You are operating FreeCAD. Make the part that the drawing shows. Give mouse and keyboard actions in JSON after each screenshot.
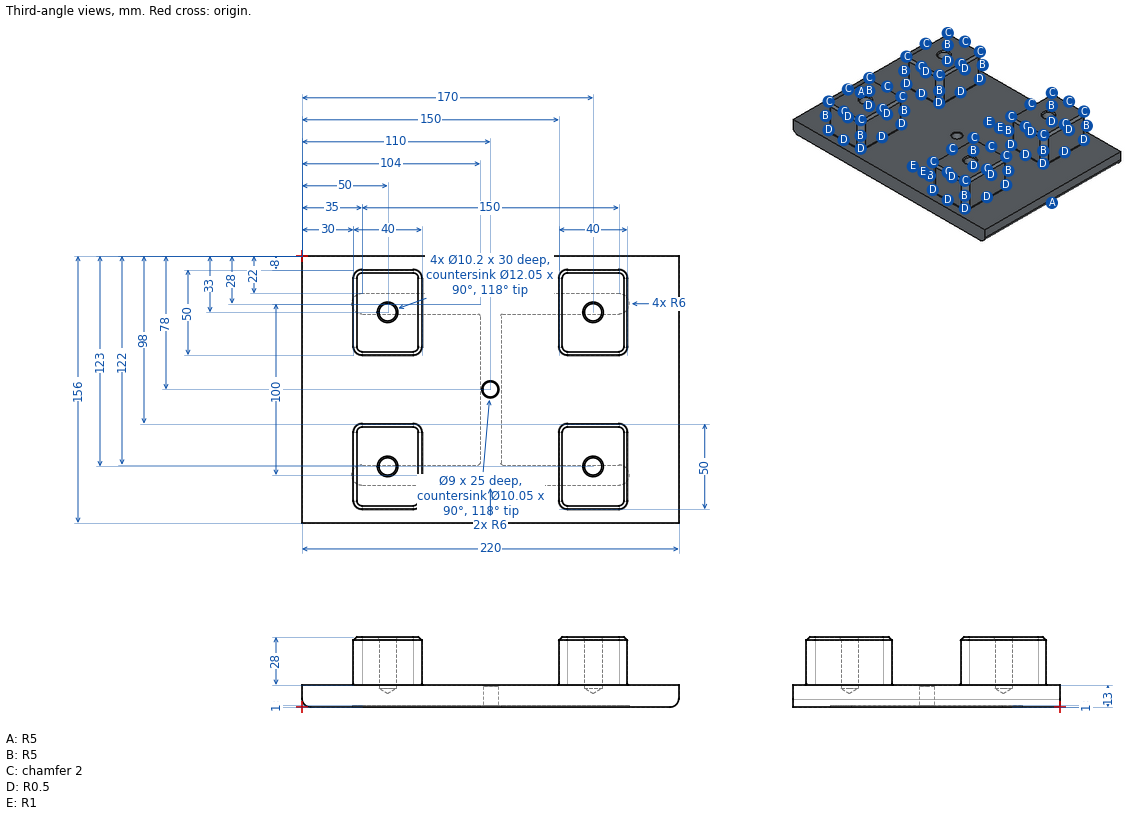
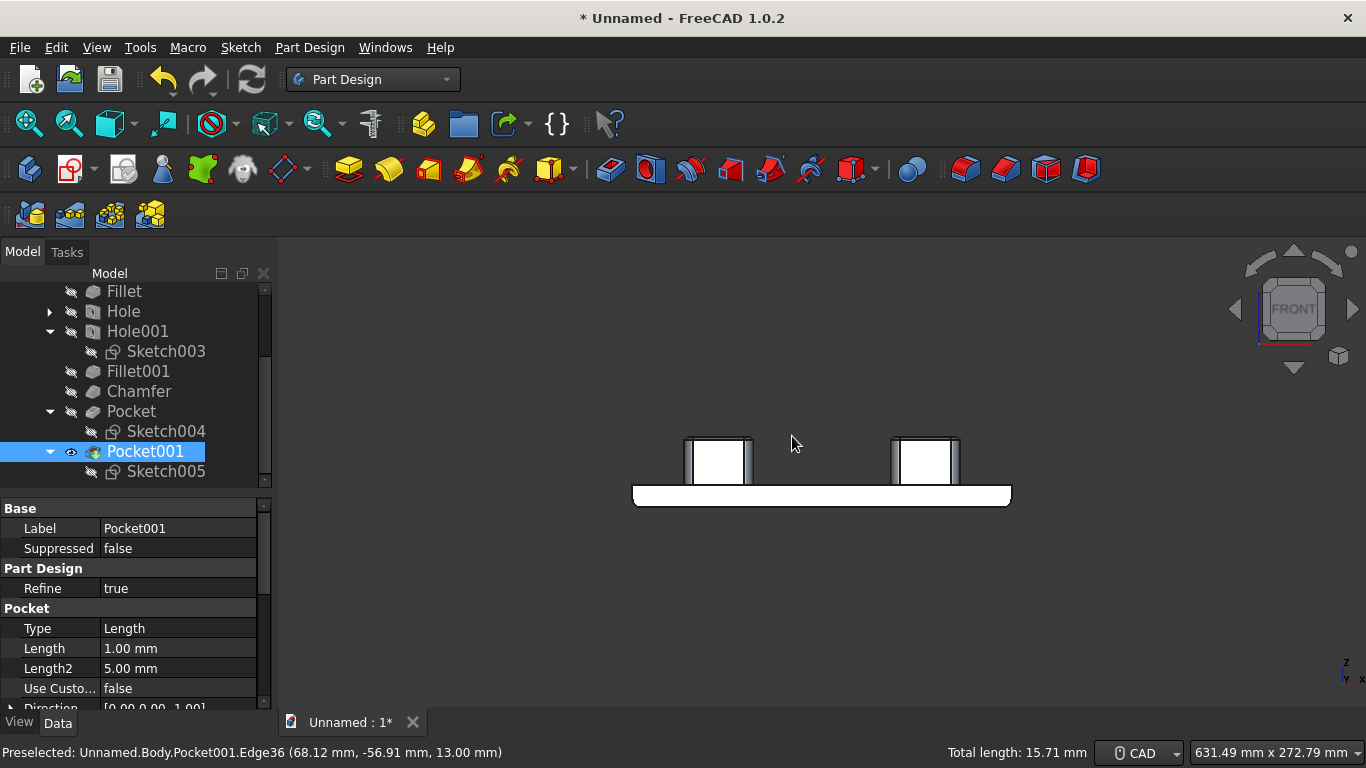
{"action": "key", "text": "v f"}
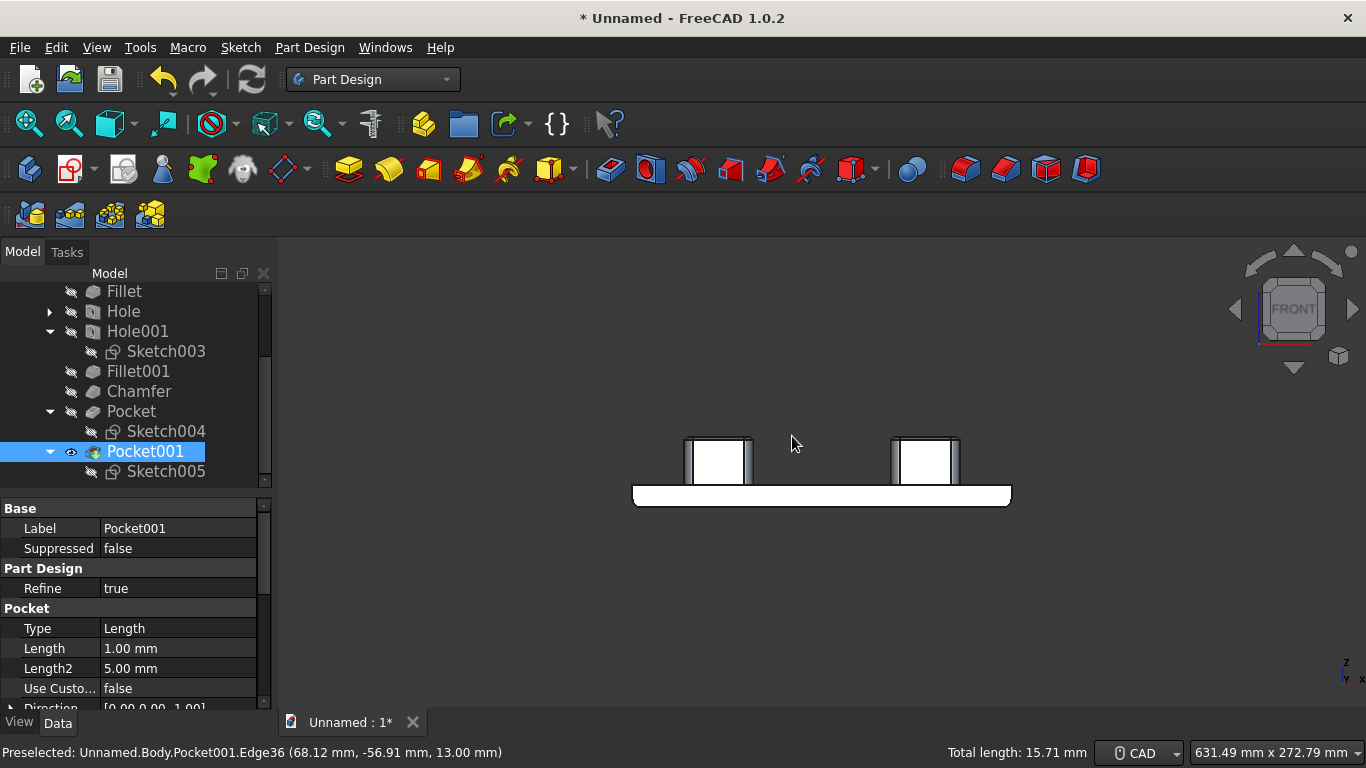
{"action": "key", "text": "3"}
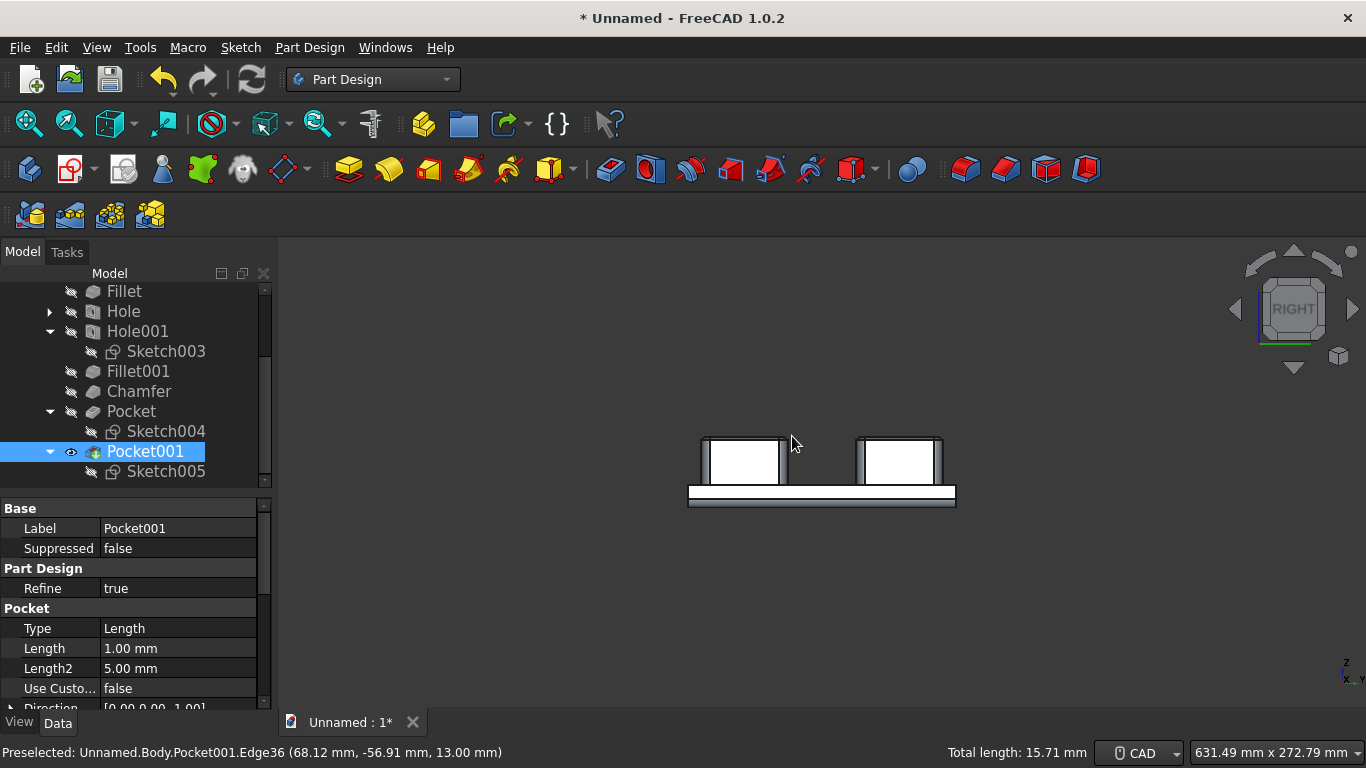
{"action": "key", "text": "v f"}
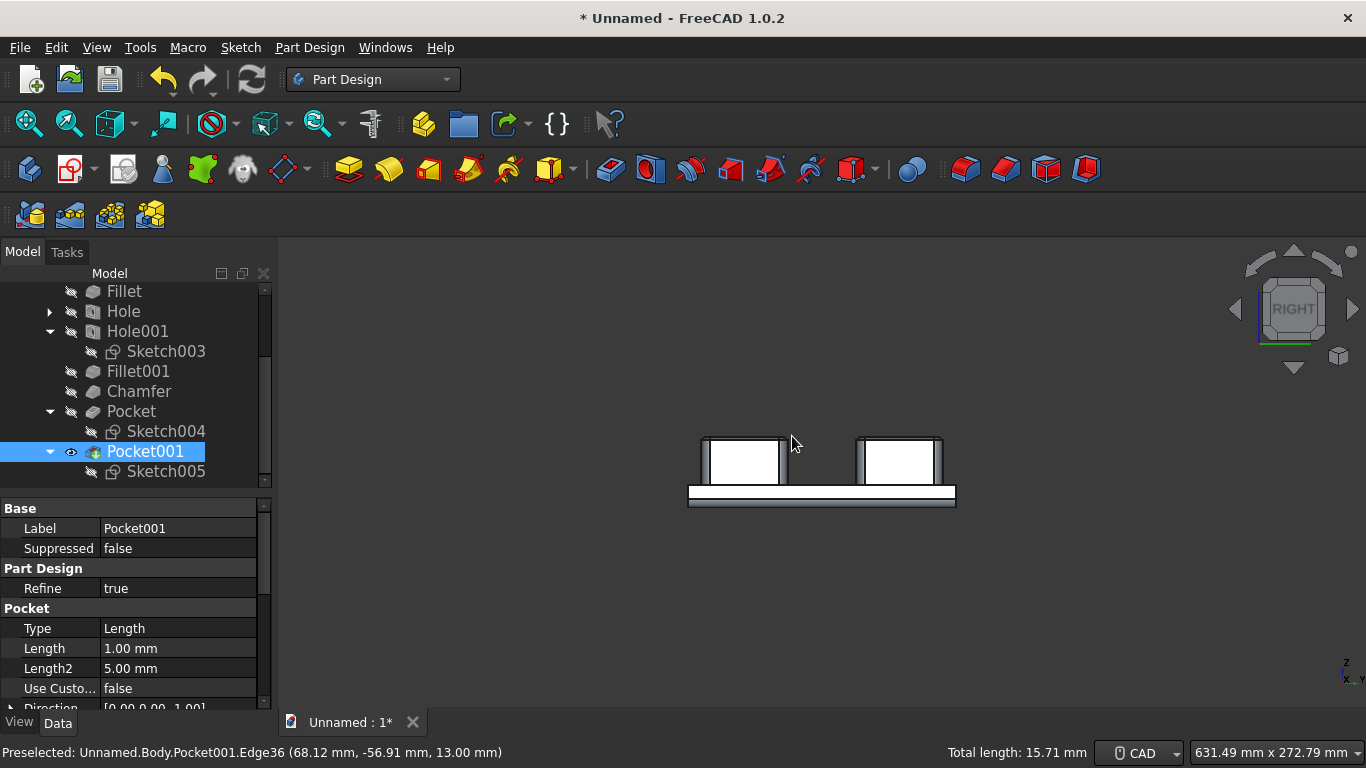
{"action": "key", "text": "5"}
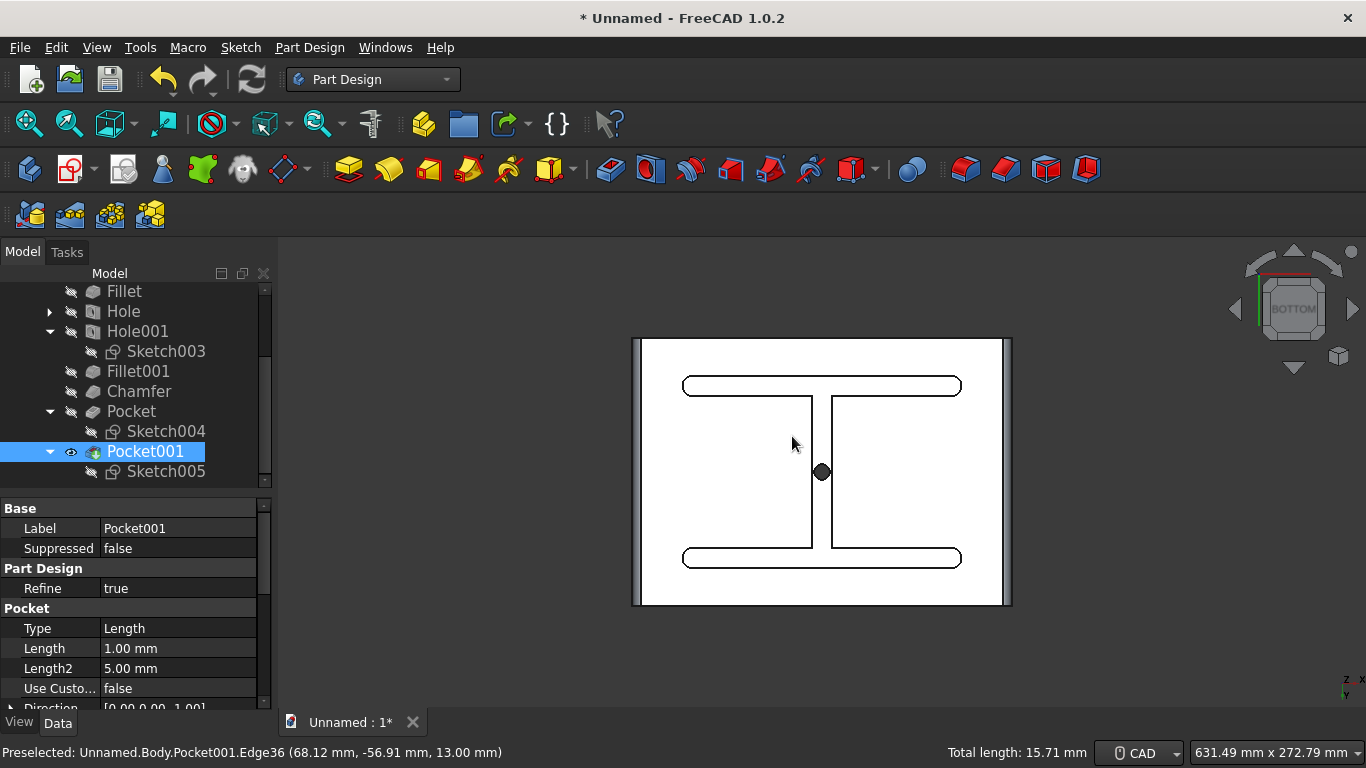
{"action": "key", "text": "4"}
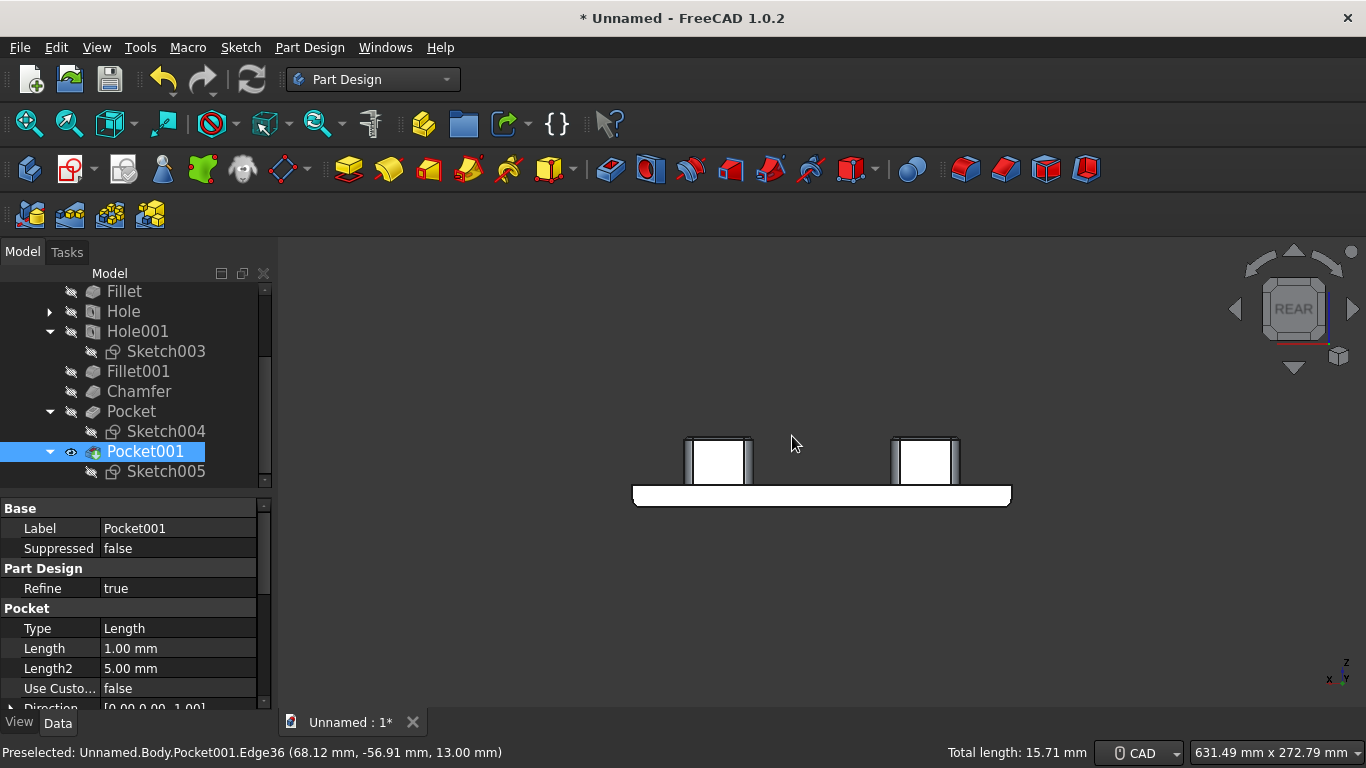
{"action": "key", "text": "v f"}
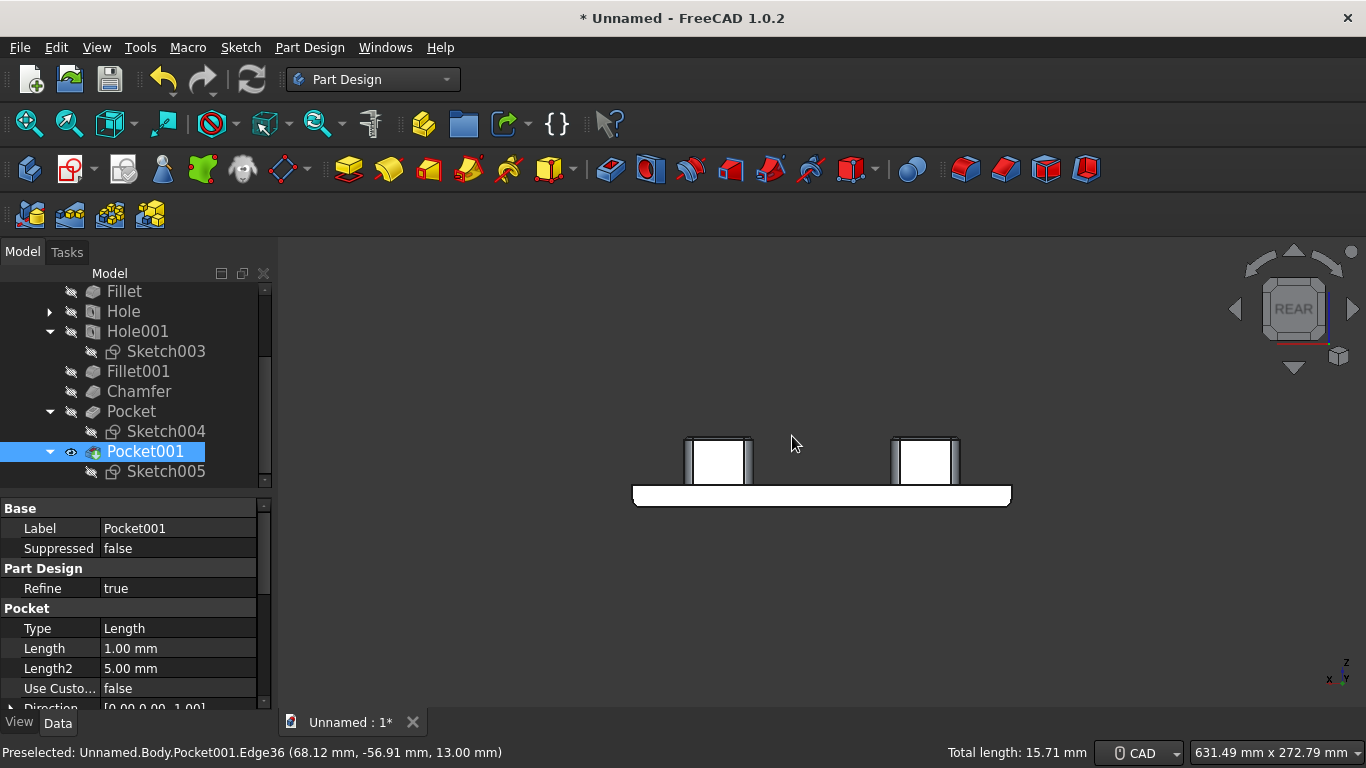
{"action": "key", "text": "6"}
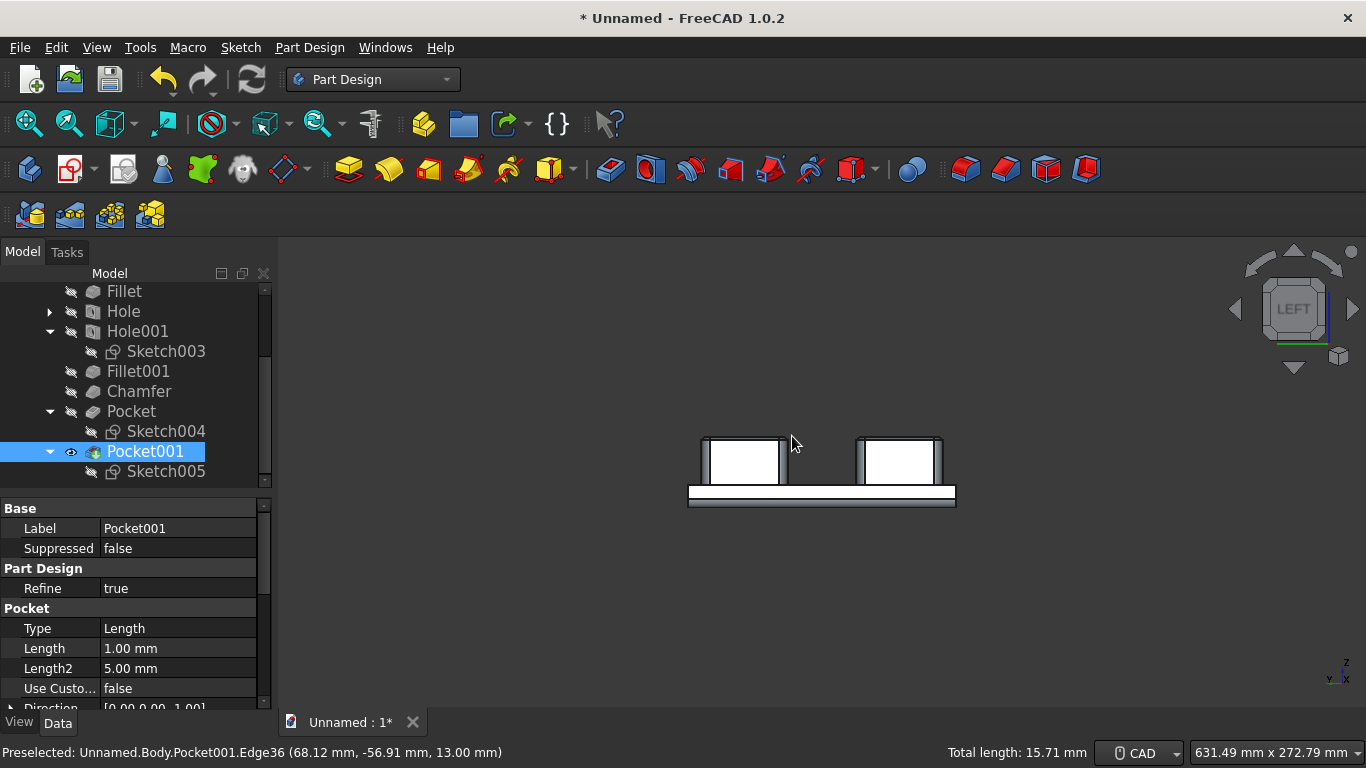
{"action": "left_click", "coordinate": [30, 124]}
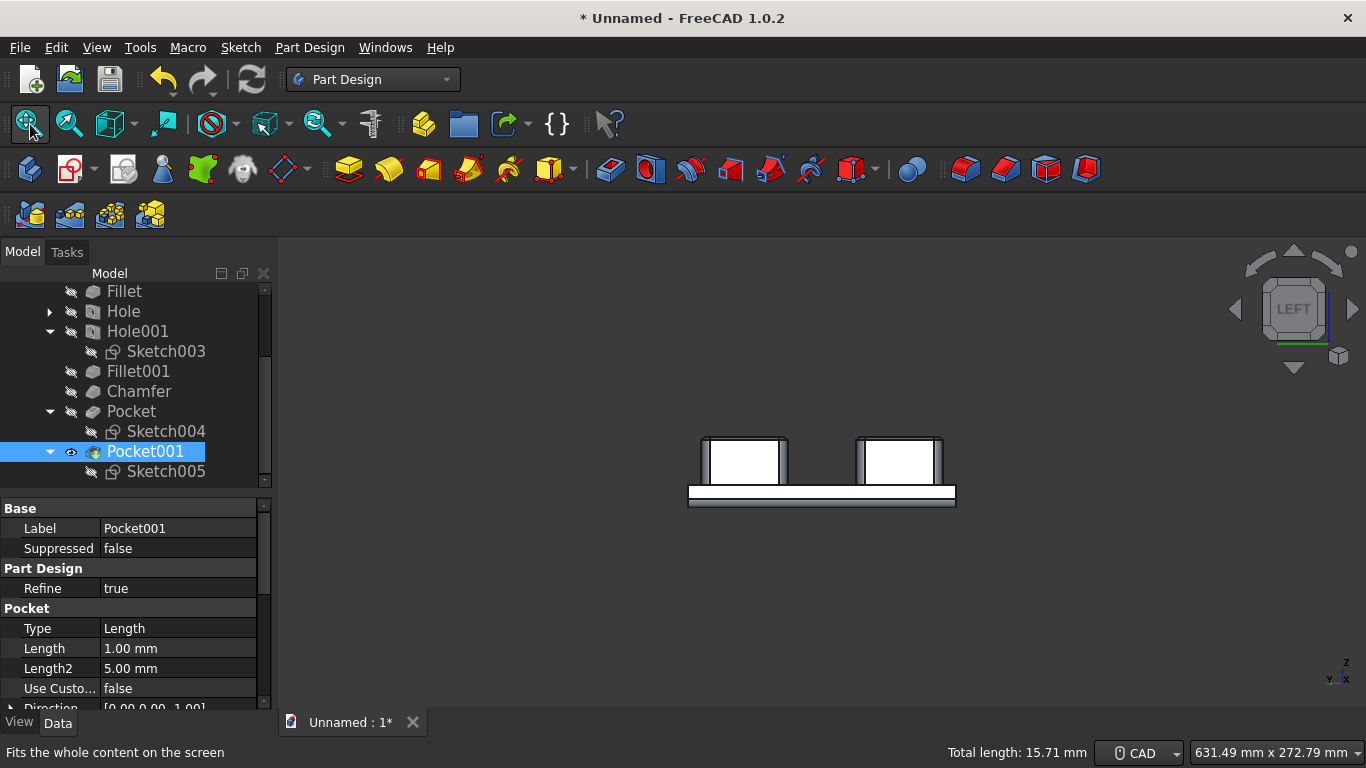
{"action": "key", "text": "v 3"}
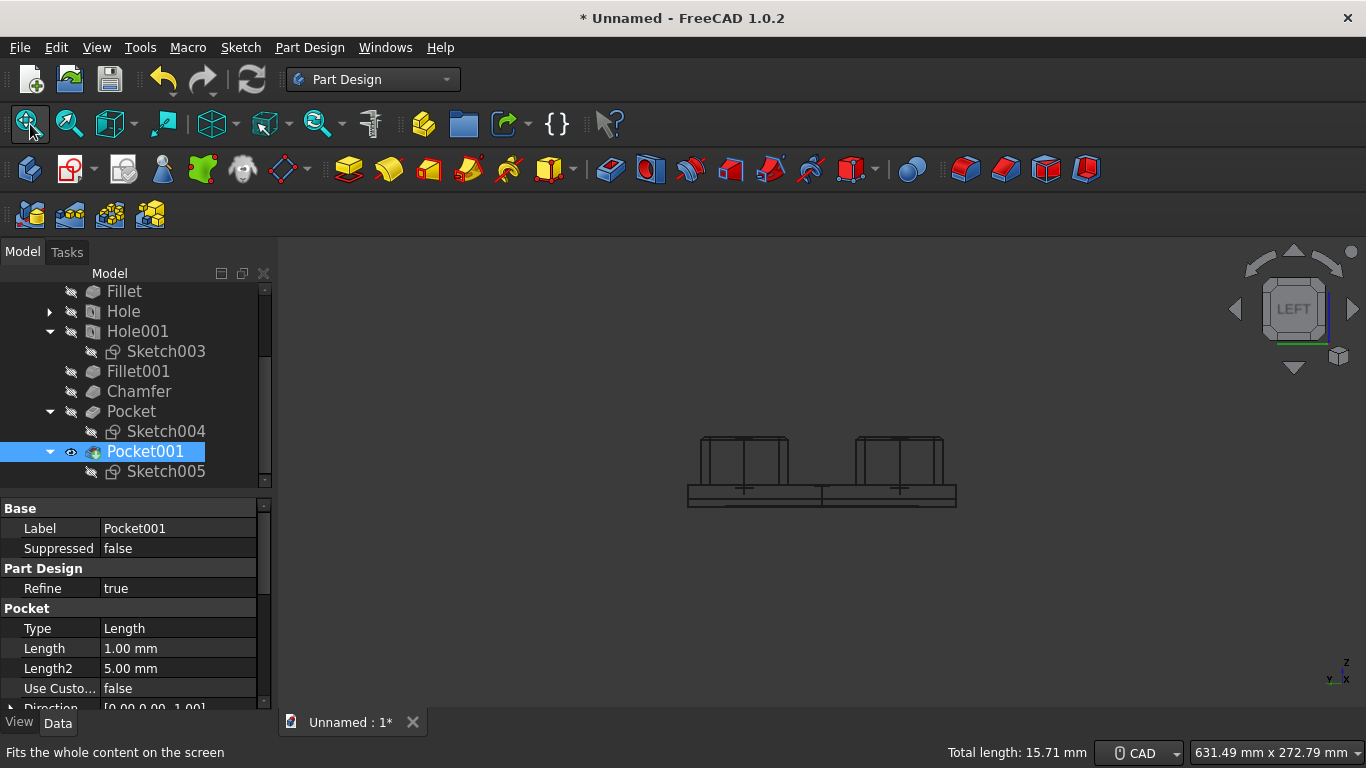
{"action": "key", "text": "0"}